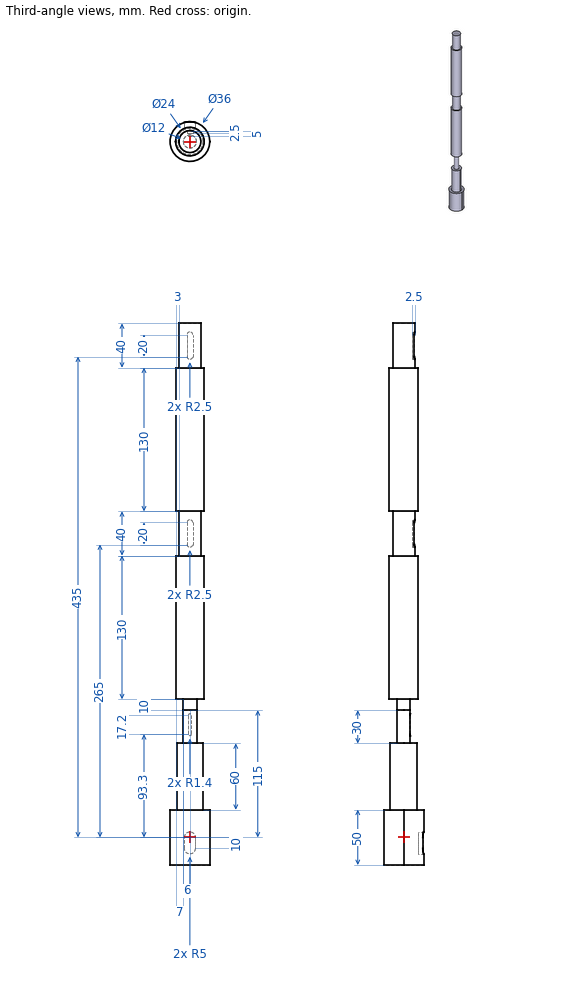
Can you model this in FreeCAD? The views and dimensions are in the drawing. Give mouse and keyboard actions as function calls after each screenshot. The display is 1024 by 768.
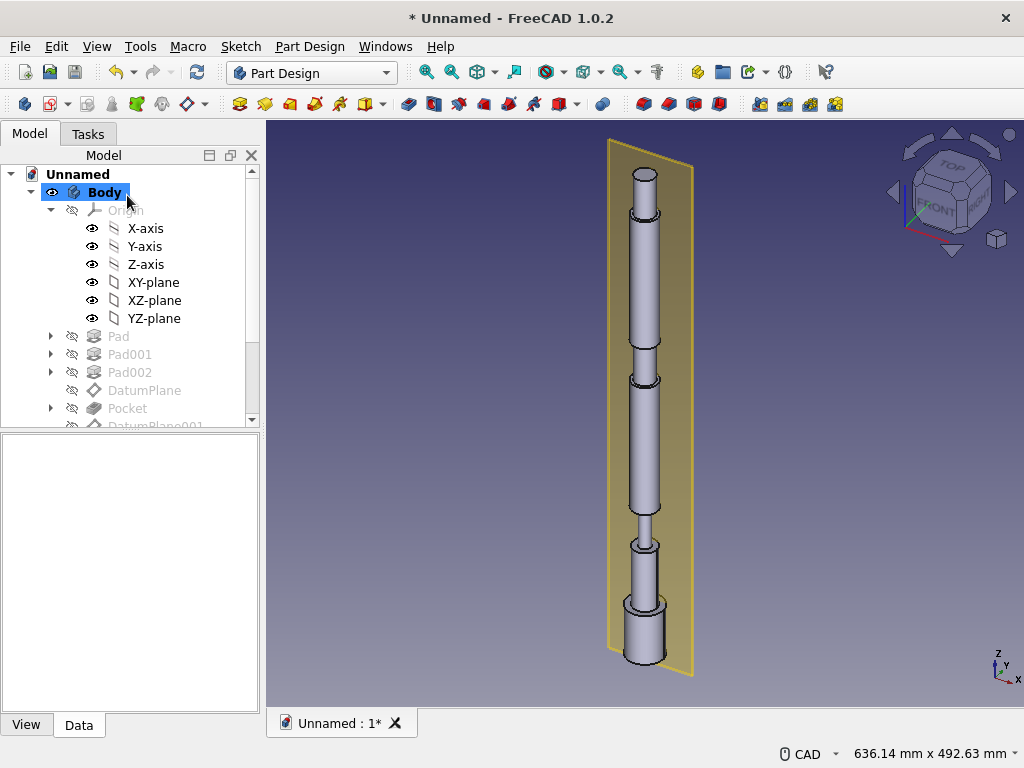
scroll(101, 296, down, 3)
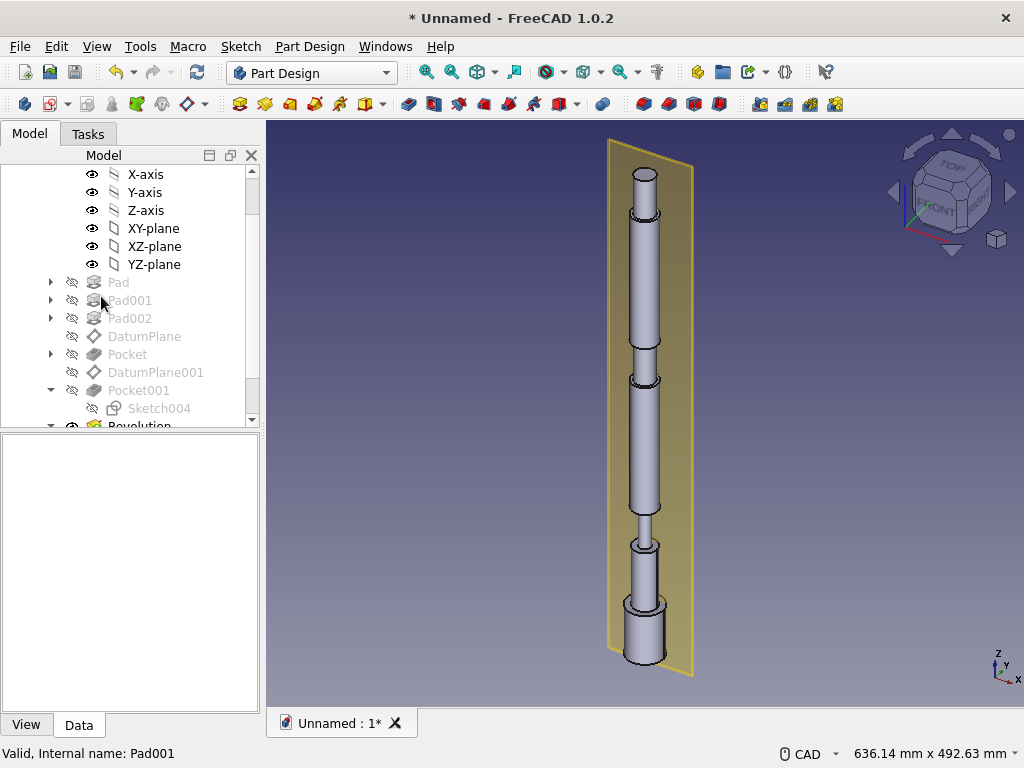
click(117, 408)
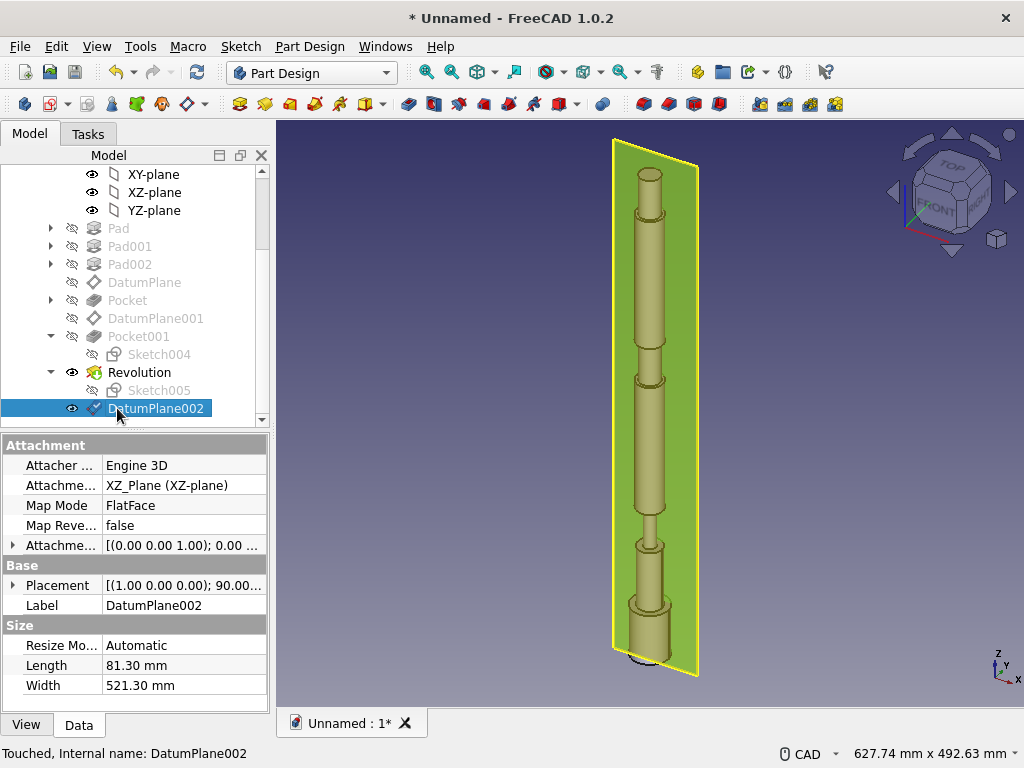
click(50, 104)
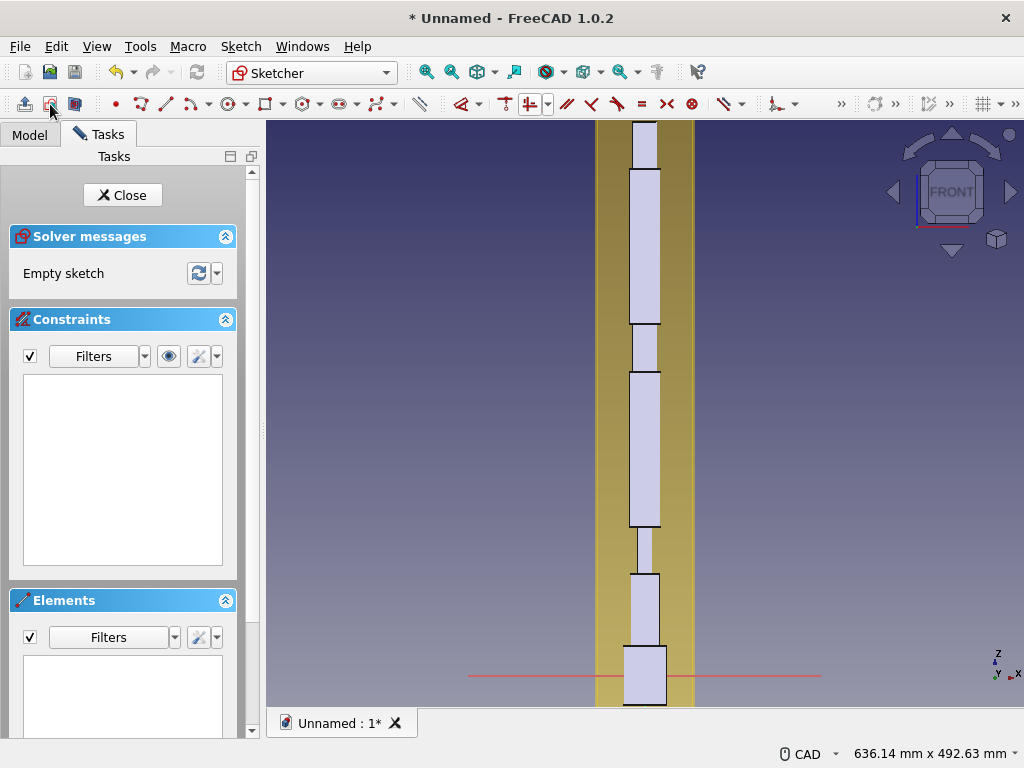
click(75, 104)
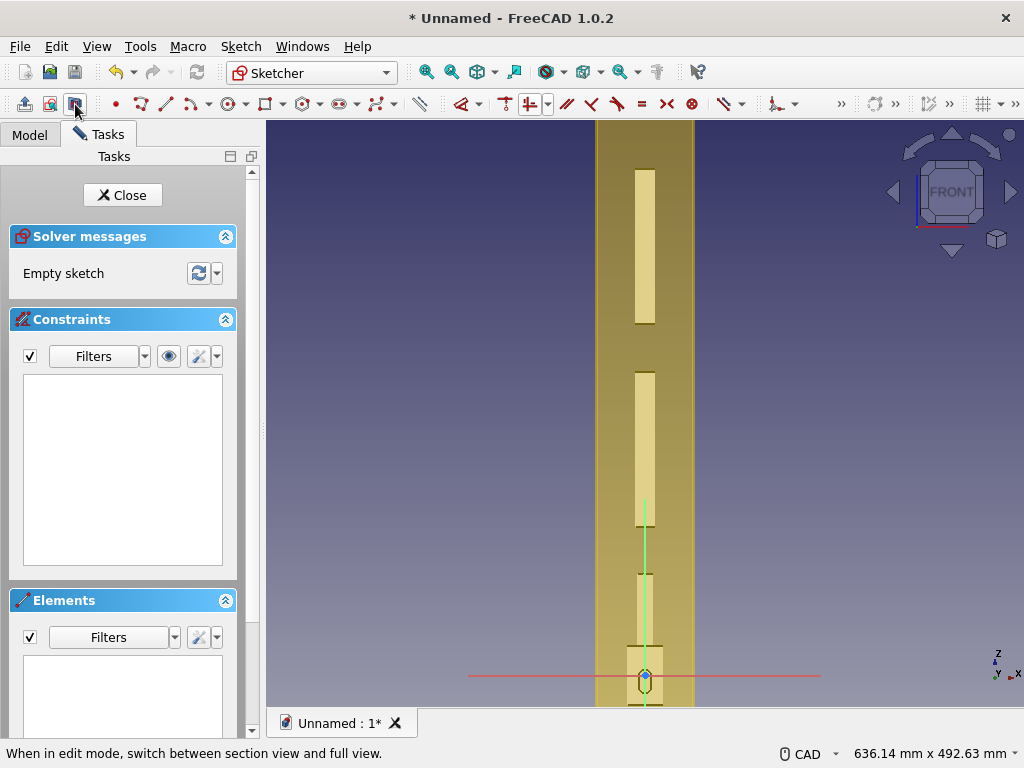
scroll(650, 343, up, 13)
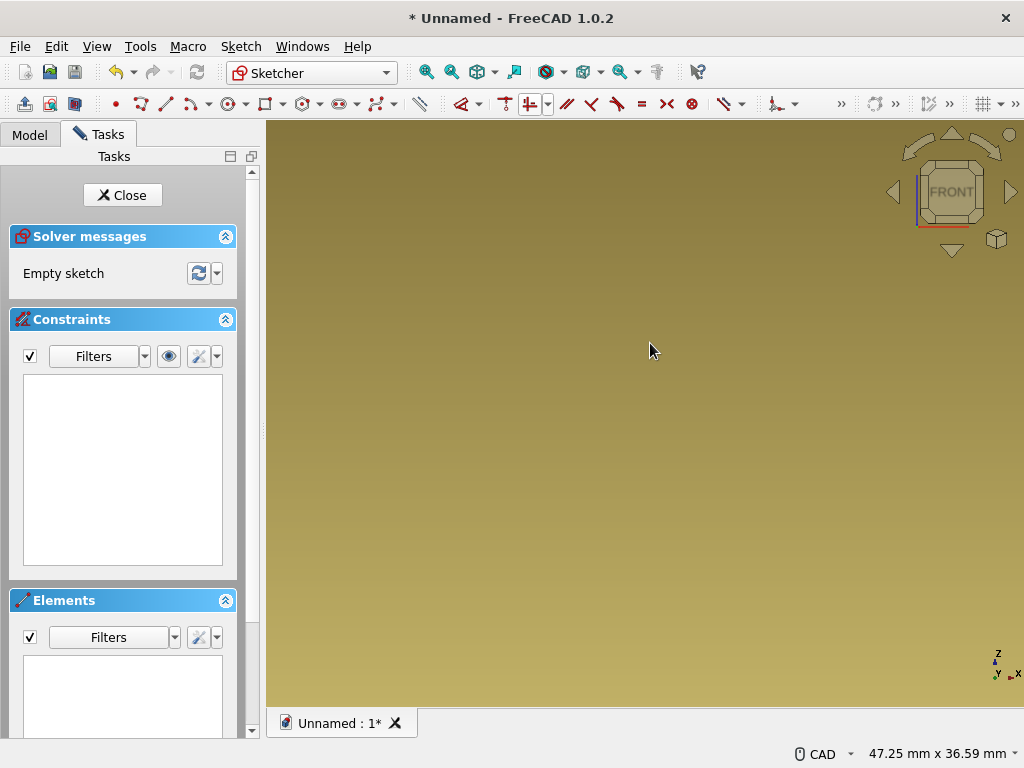
click(338, 104)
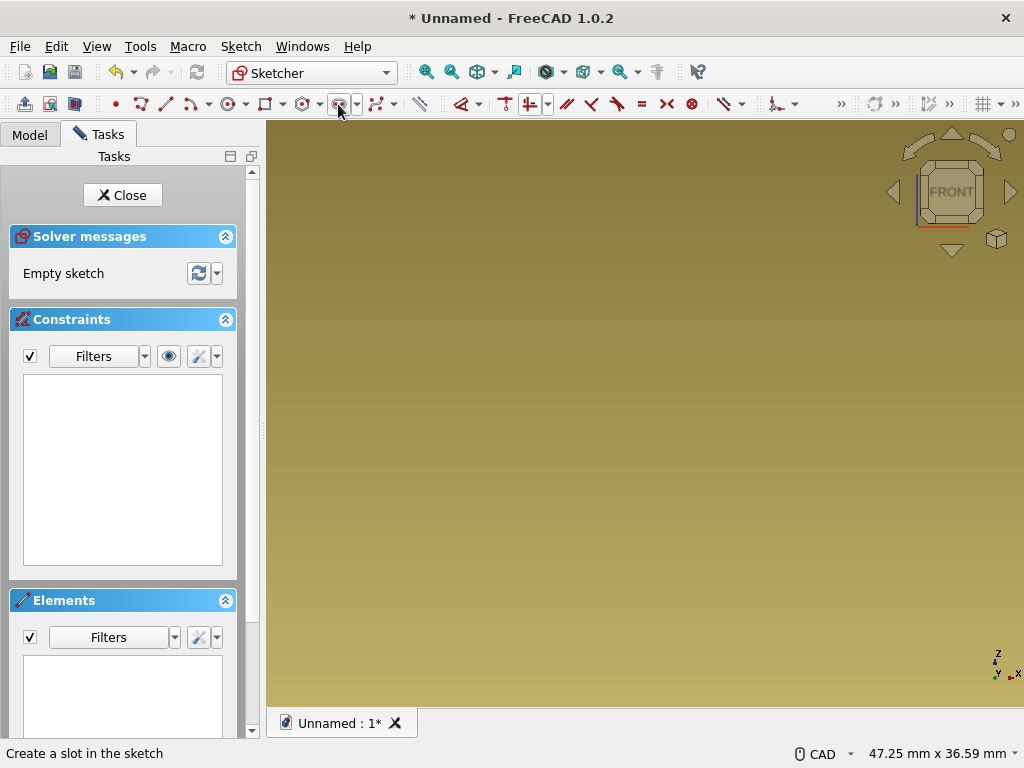
click(576, 566)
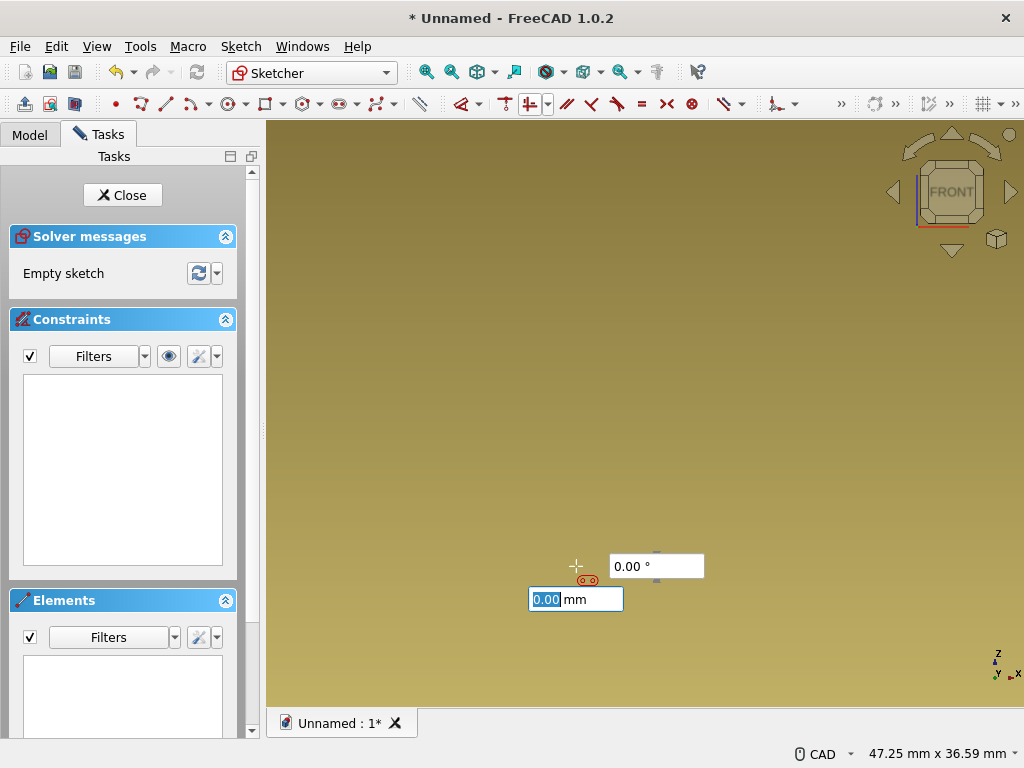
click(585, 245)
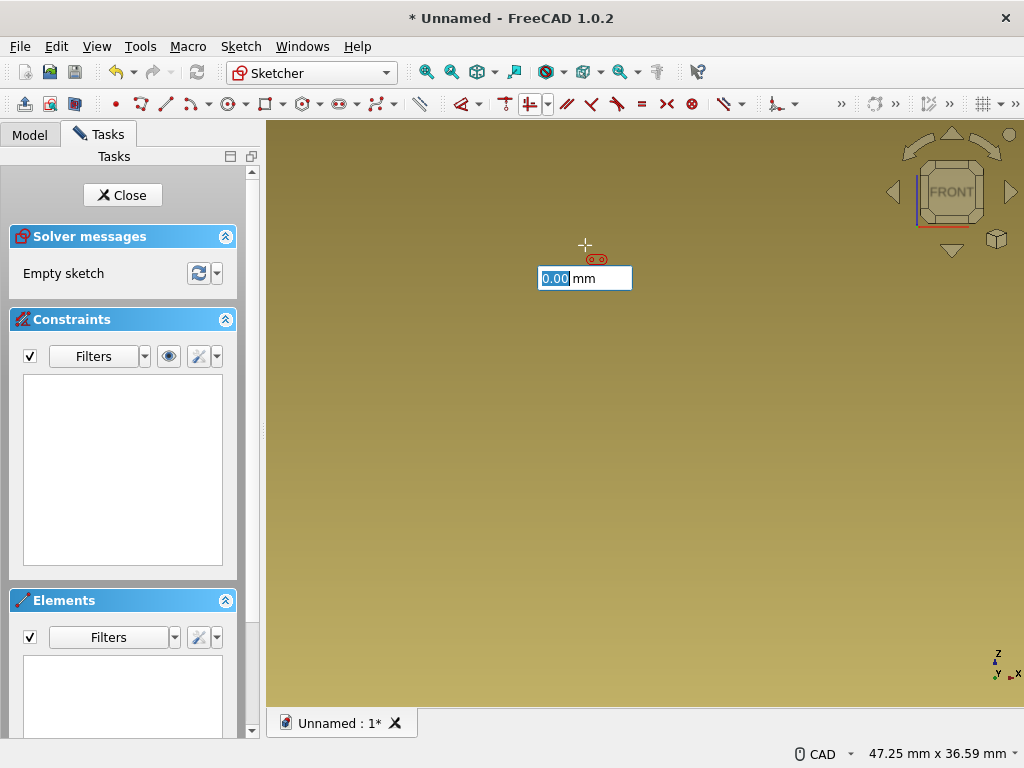
click(616, 405)
key(Escape)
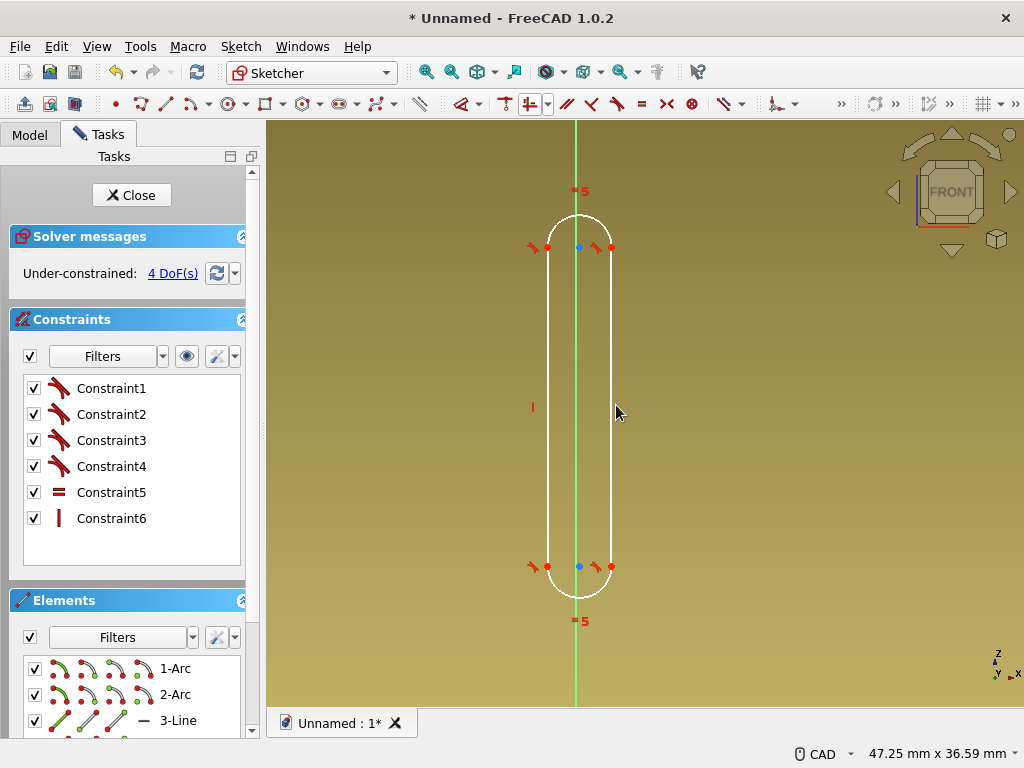
click(580, 566)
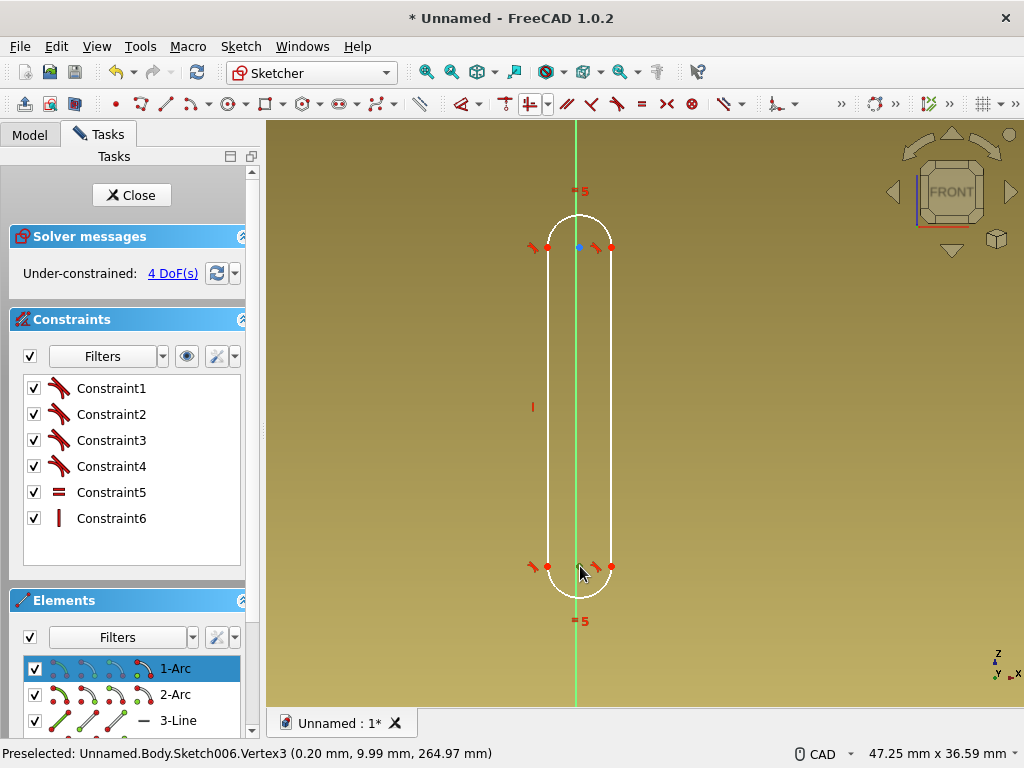
click(576, 641)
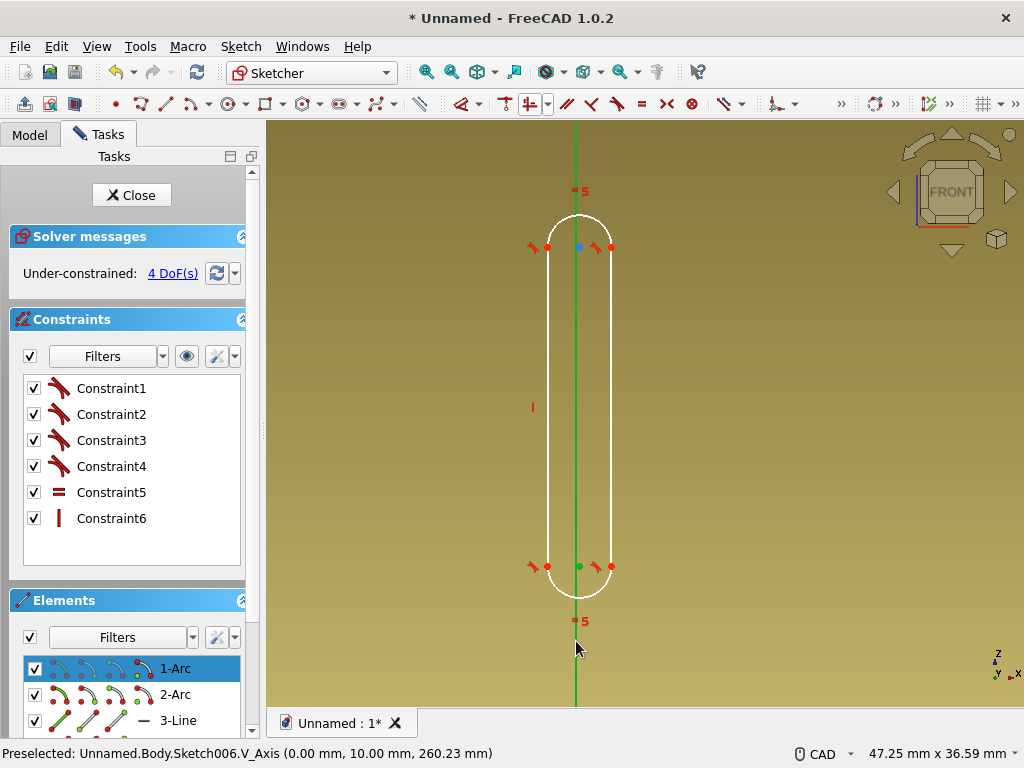
click(505, 104)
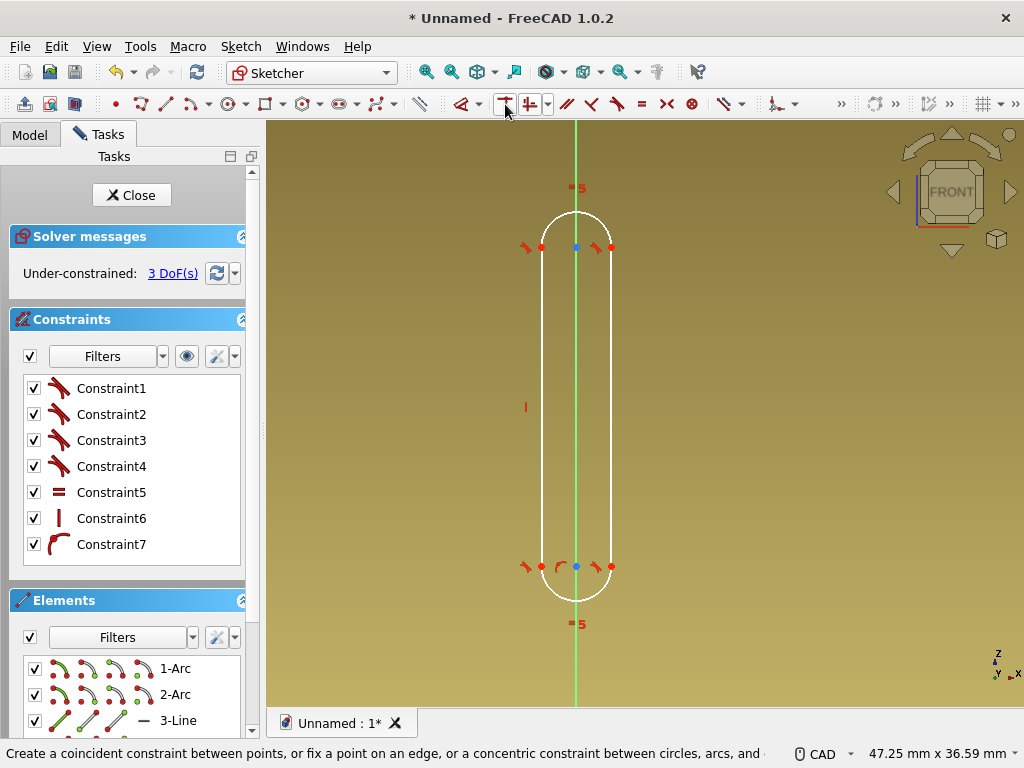
click(460, 104)